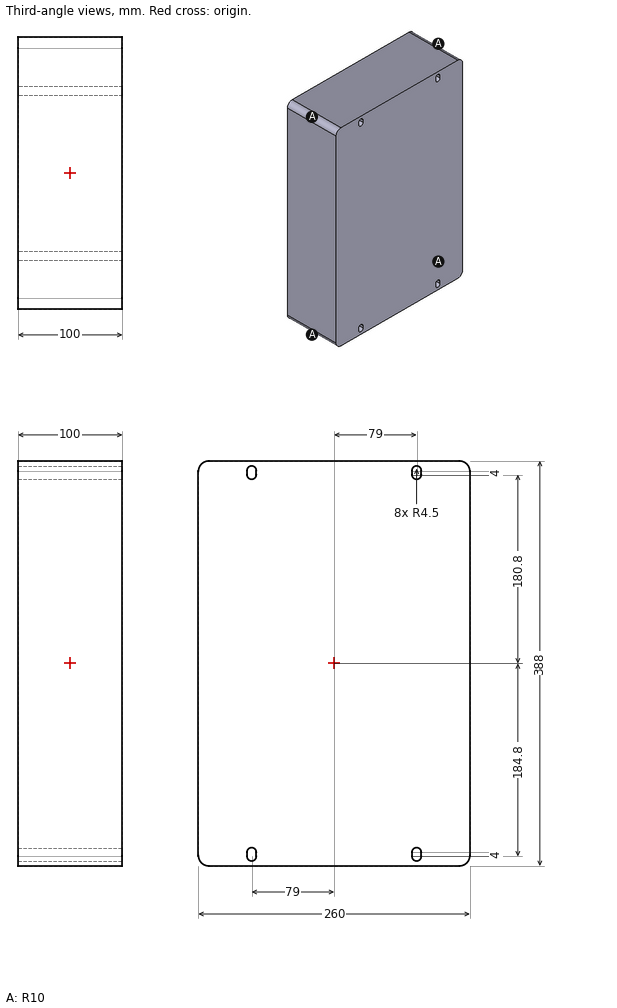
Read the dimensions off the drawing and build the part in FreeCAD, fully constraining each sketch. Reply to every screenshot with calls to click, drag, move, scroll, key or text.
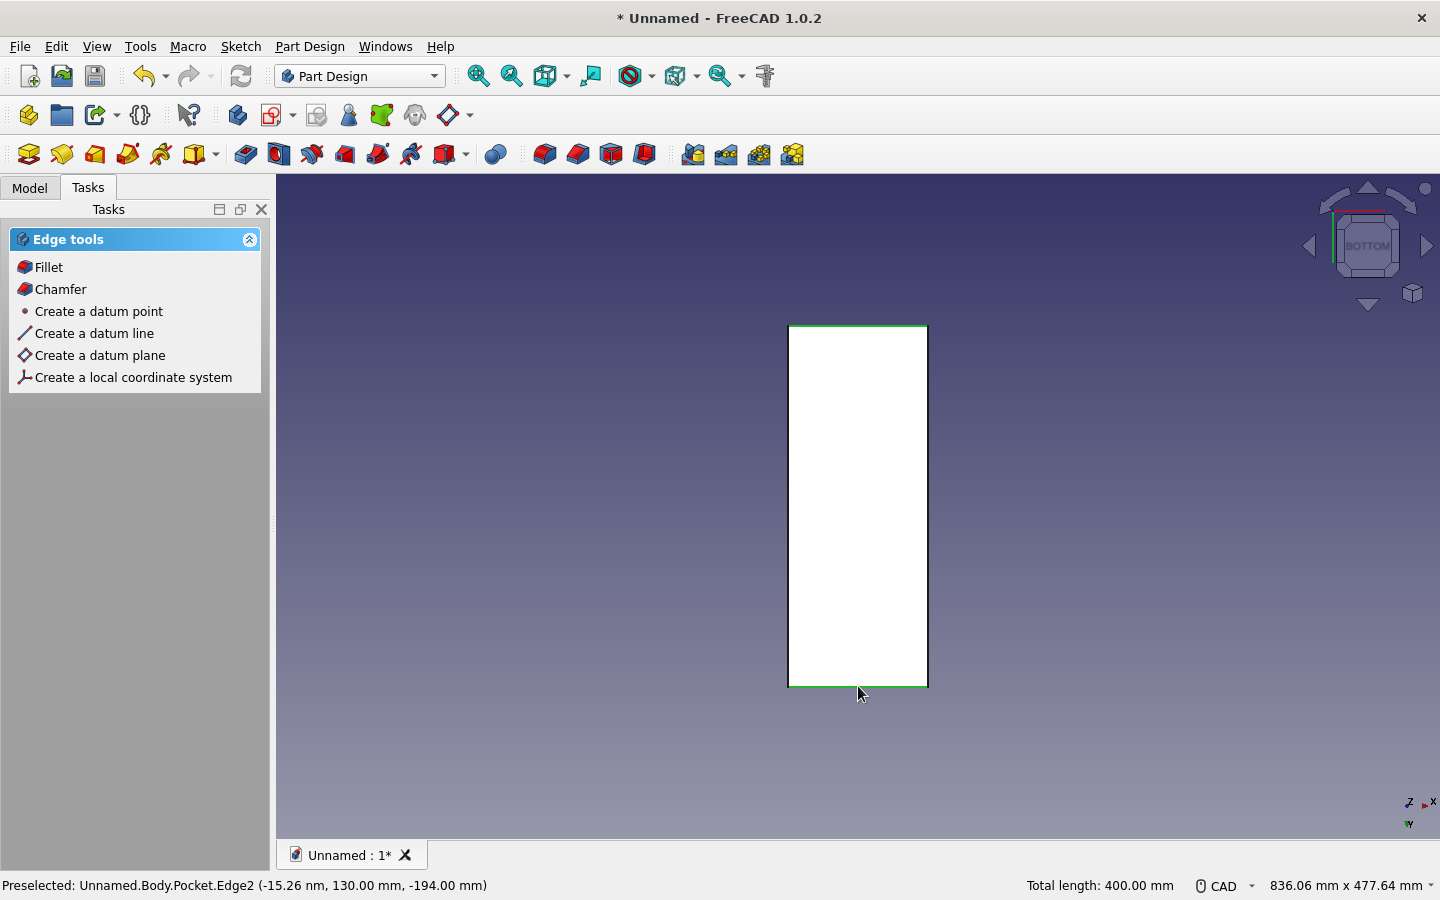
click(545, 154)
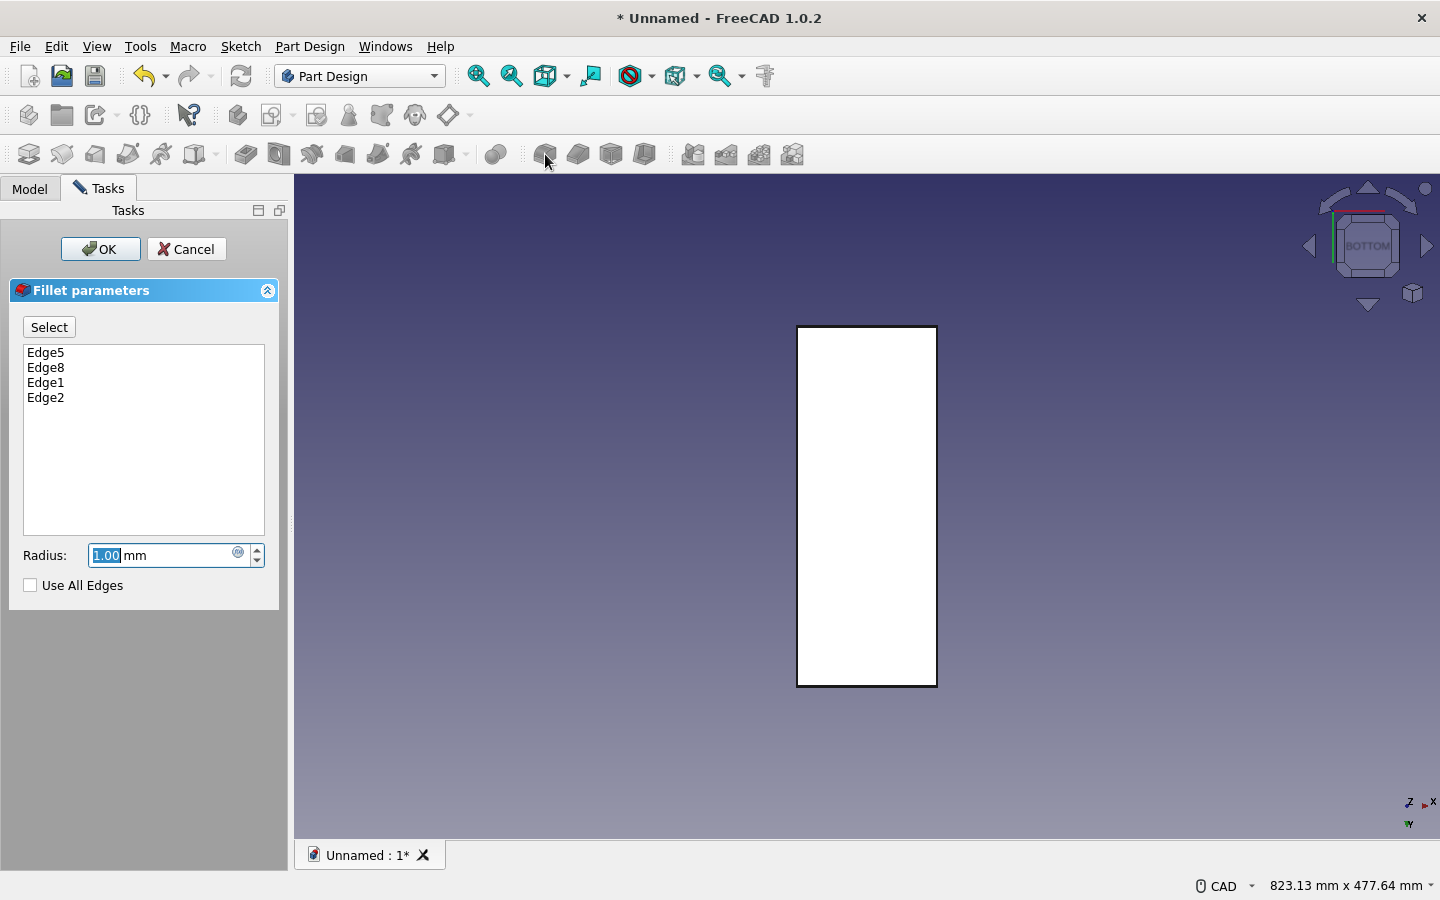
text(10)
key(Tab)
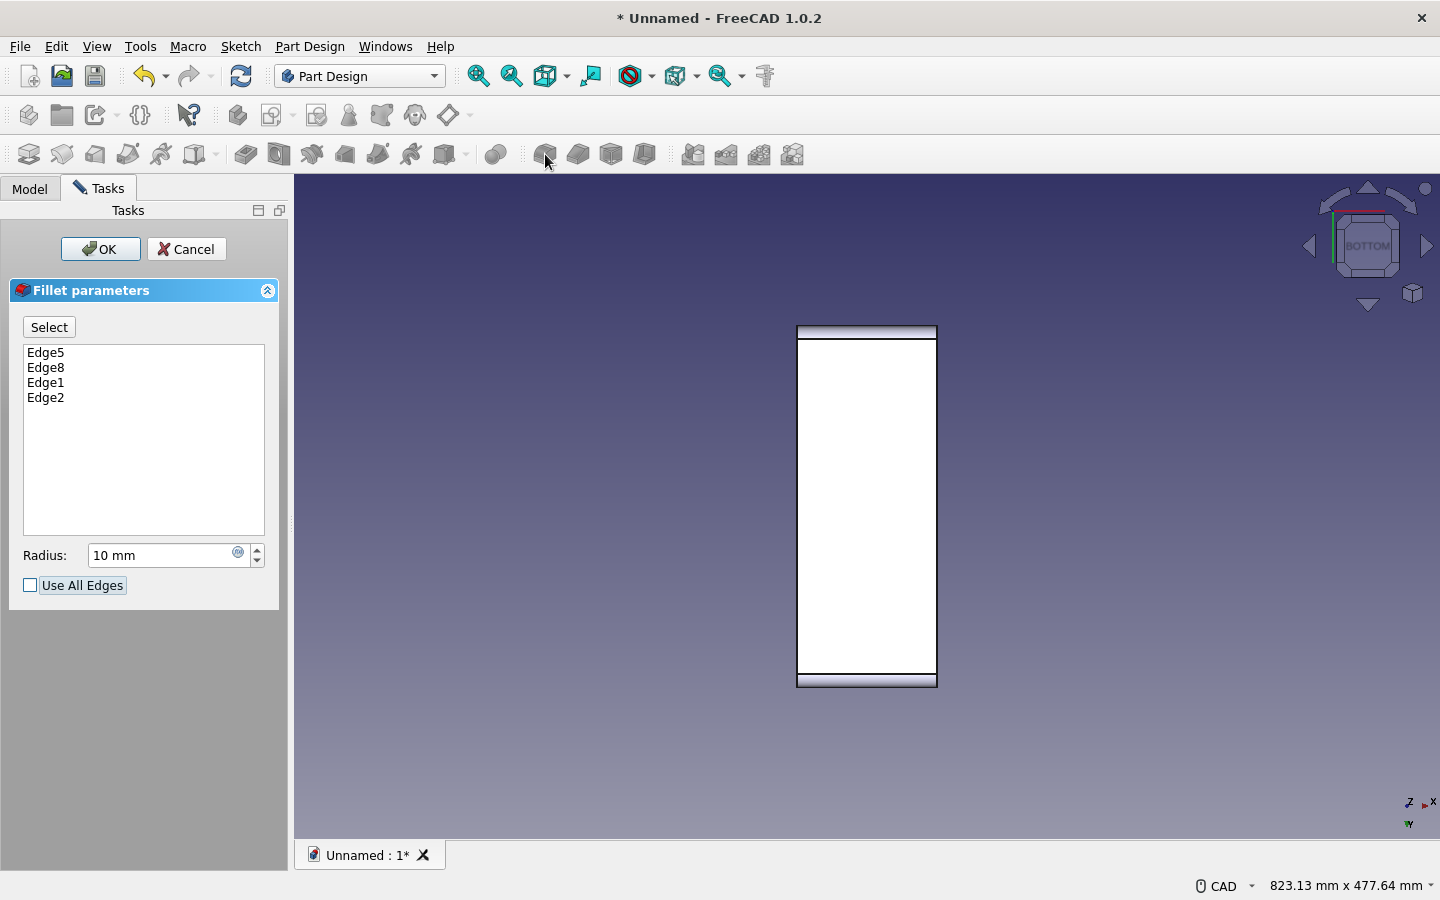
click(101, 249)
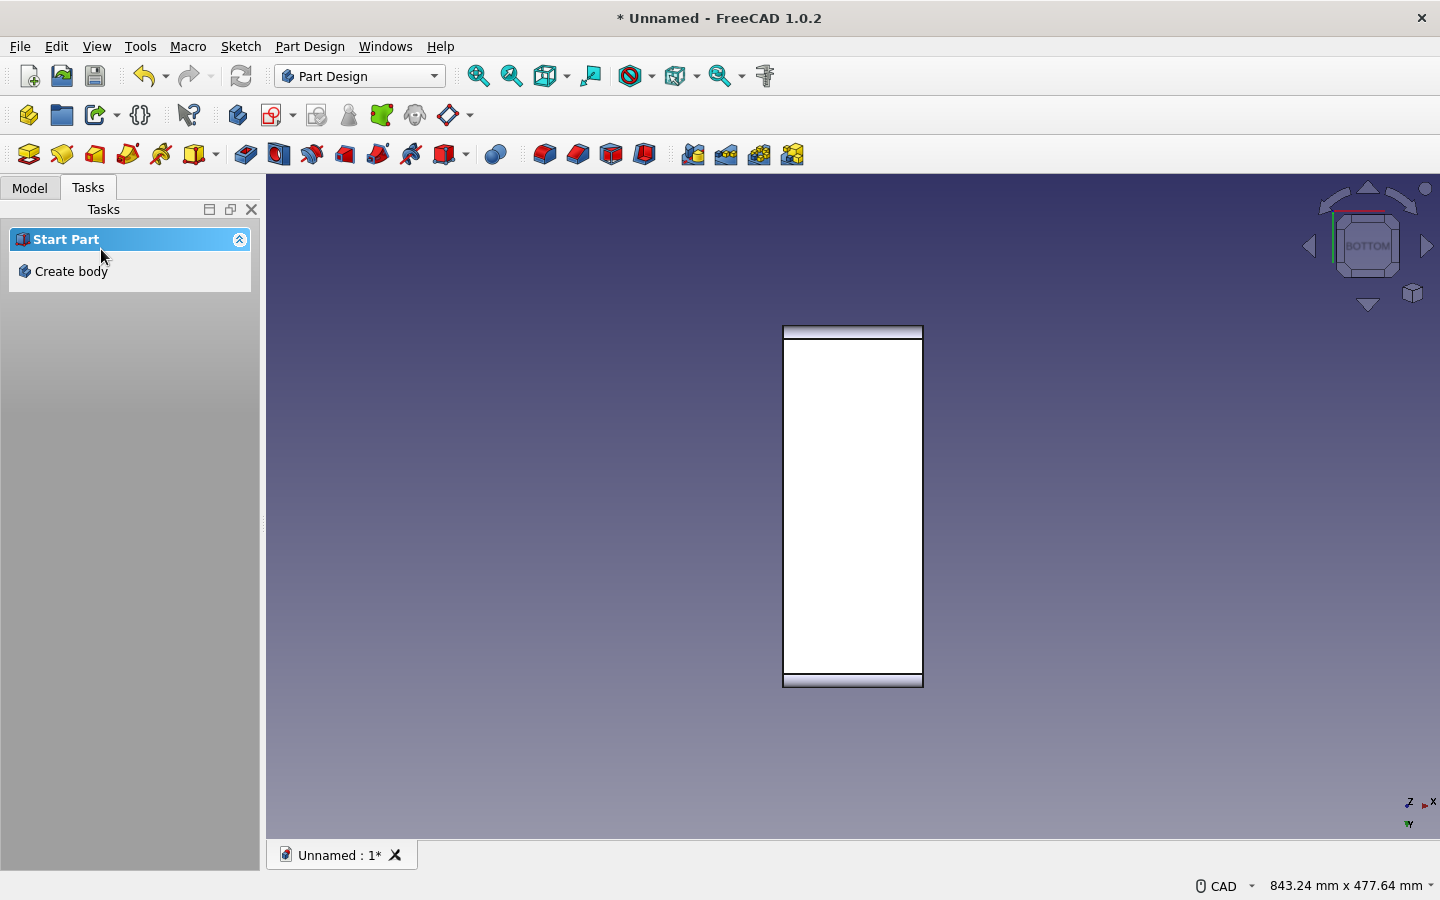
key(0)